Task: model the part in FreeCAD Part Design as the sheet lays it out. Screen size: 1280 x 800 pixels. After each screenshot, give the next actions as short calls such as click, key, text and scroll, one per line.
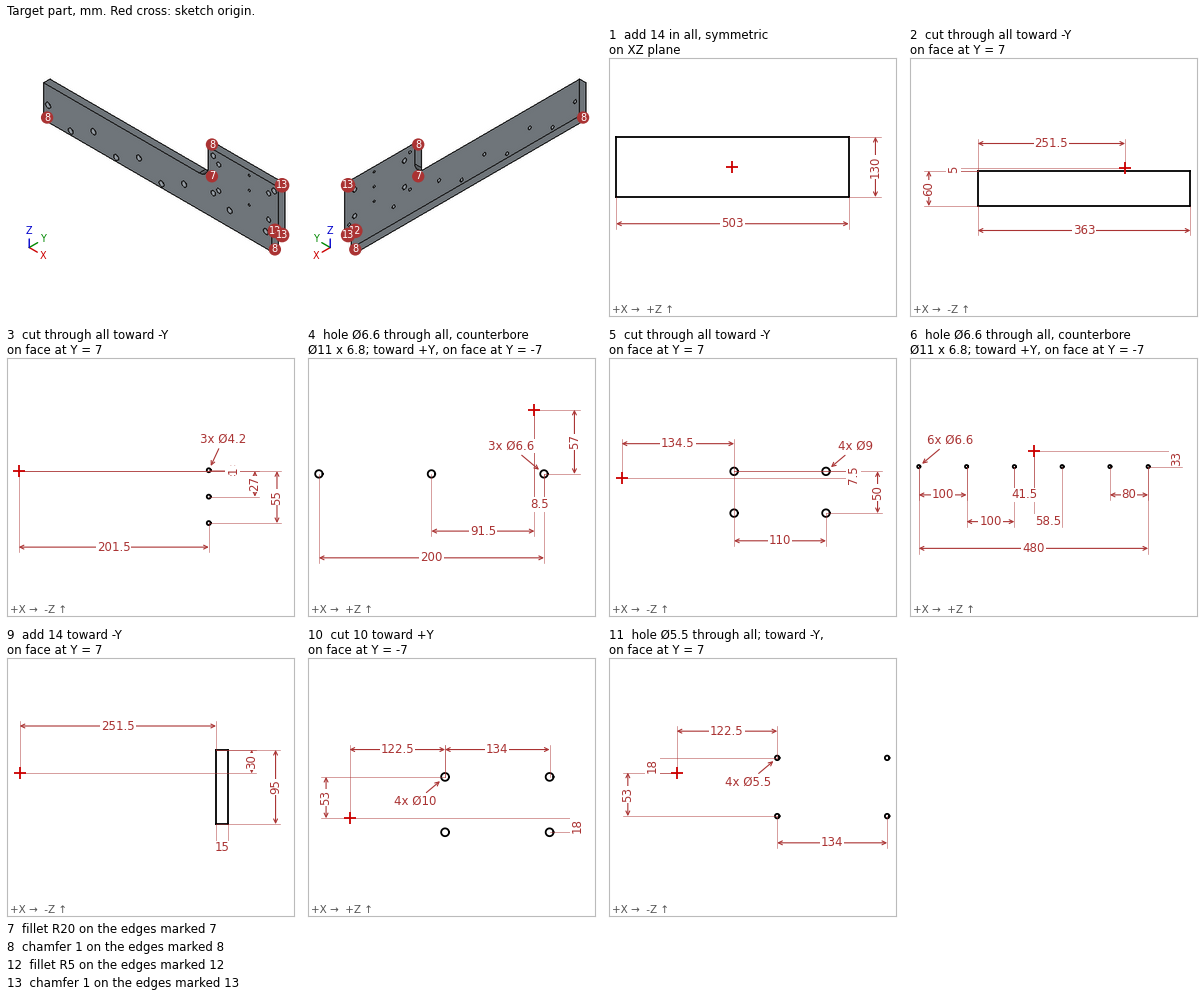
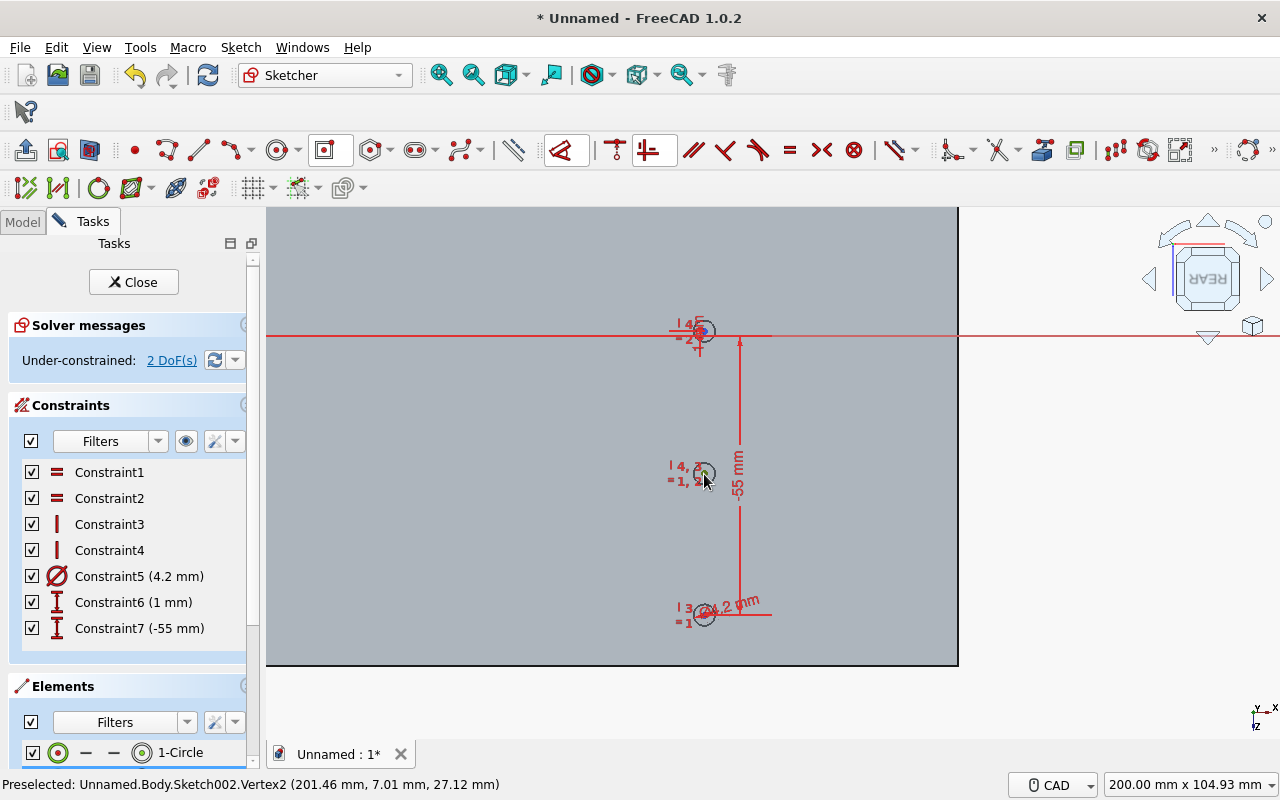
key(i)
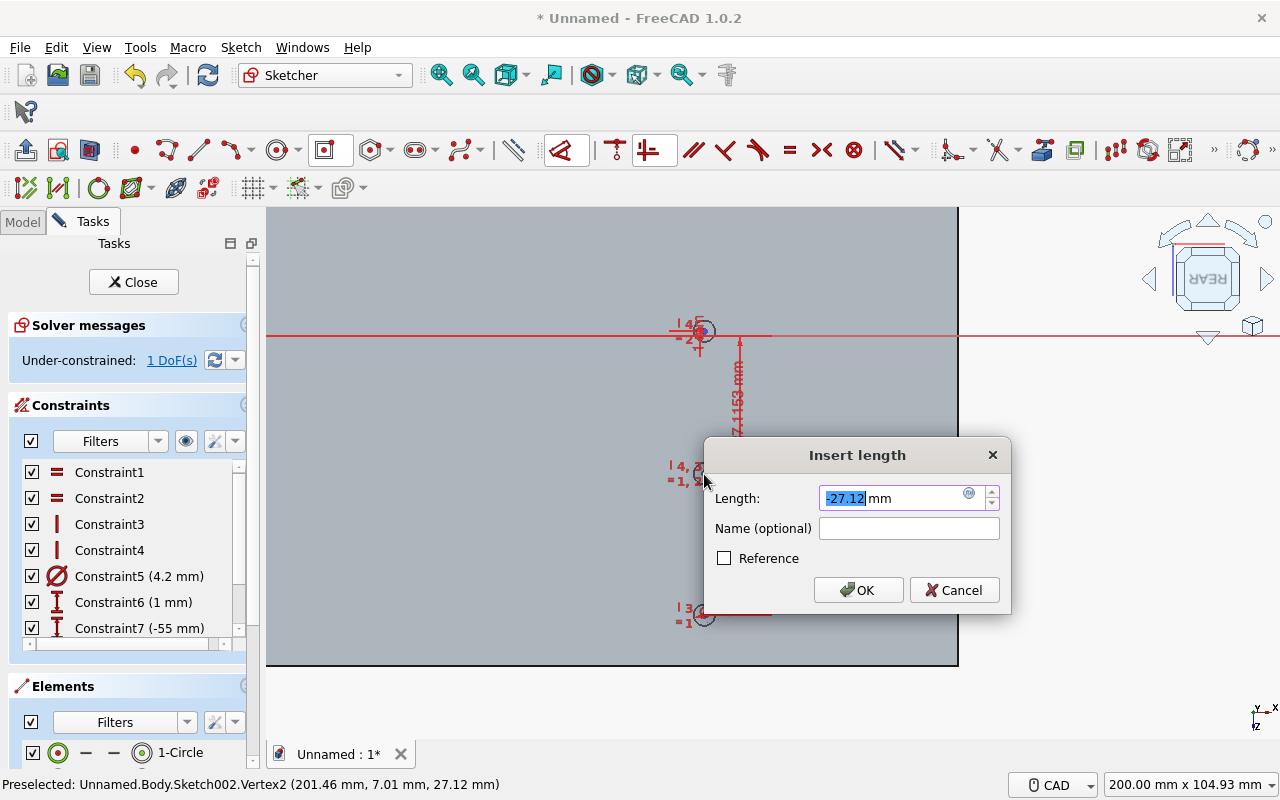
text(-27)
key(Return)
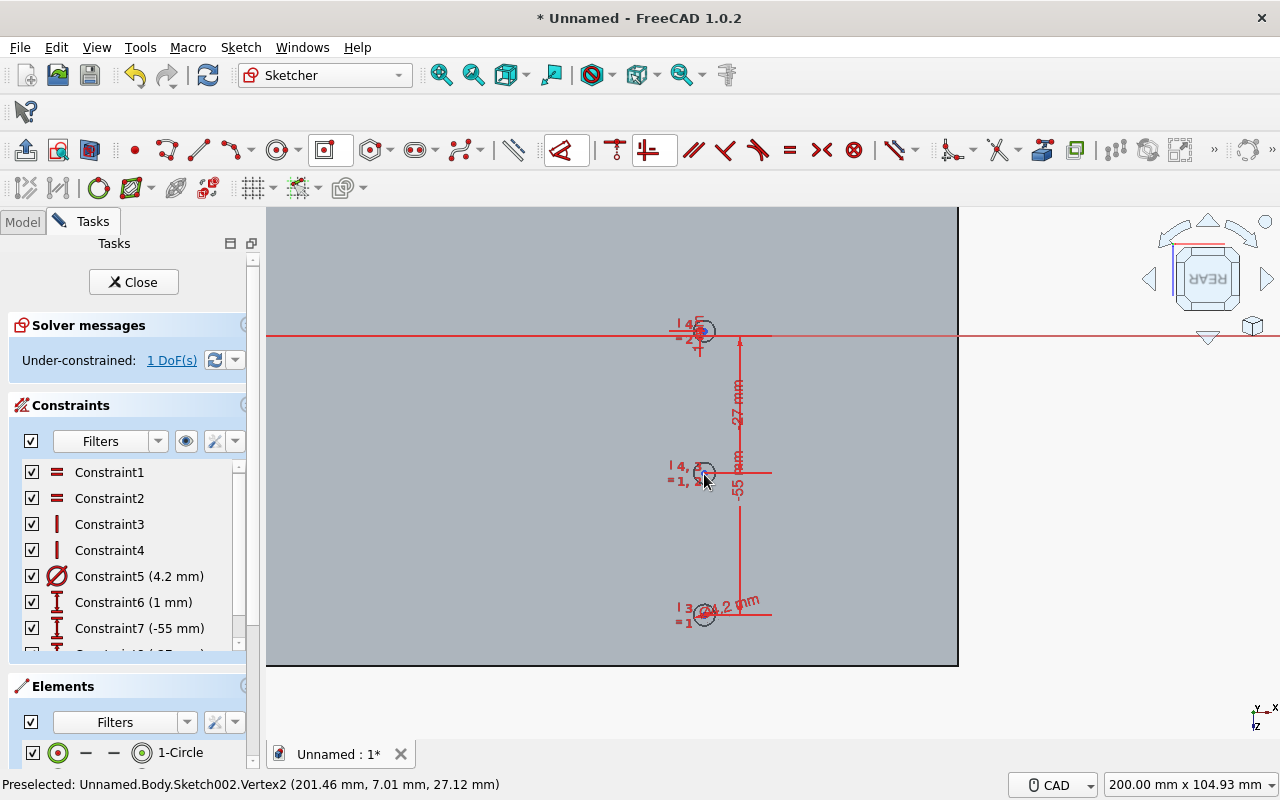
click(704, 615)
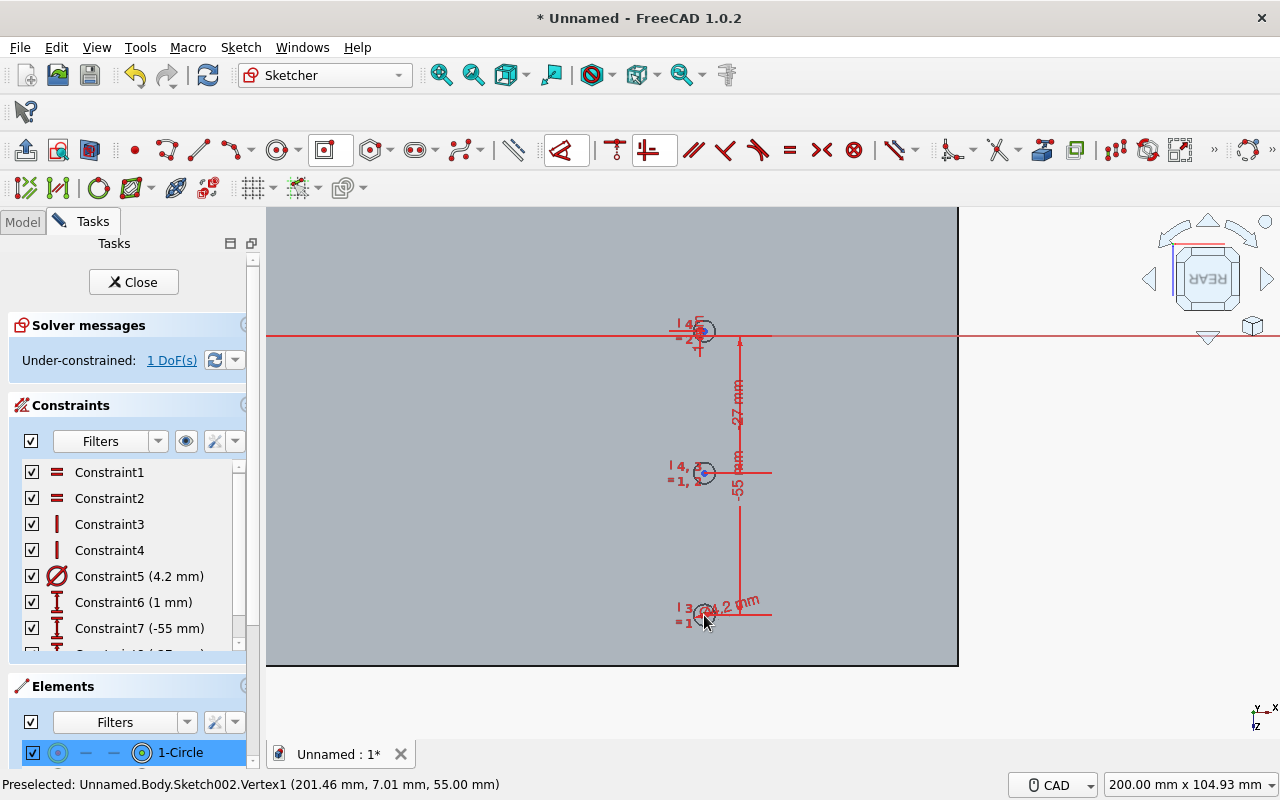
click(584, 150)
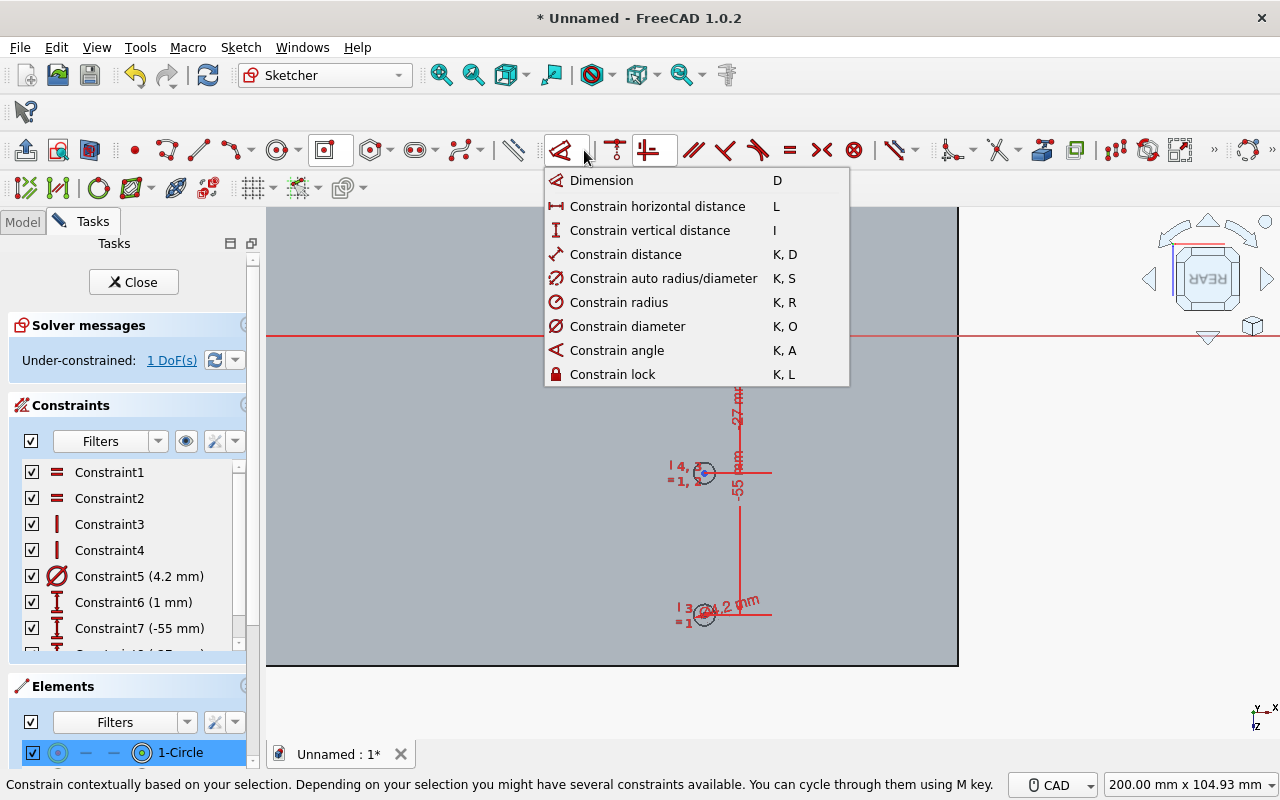
click(697, 206)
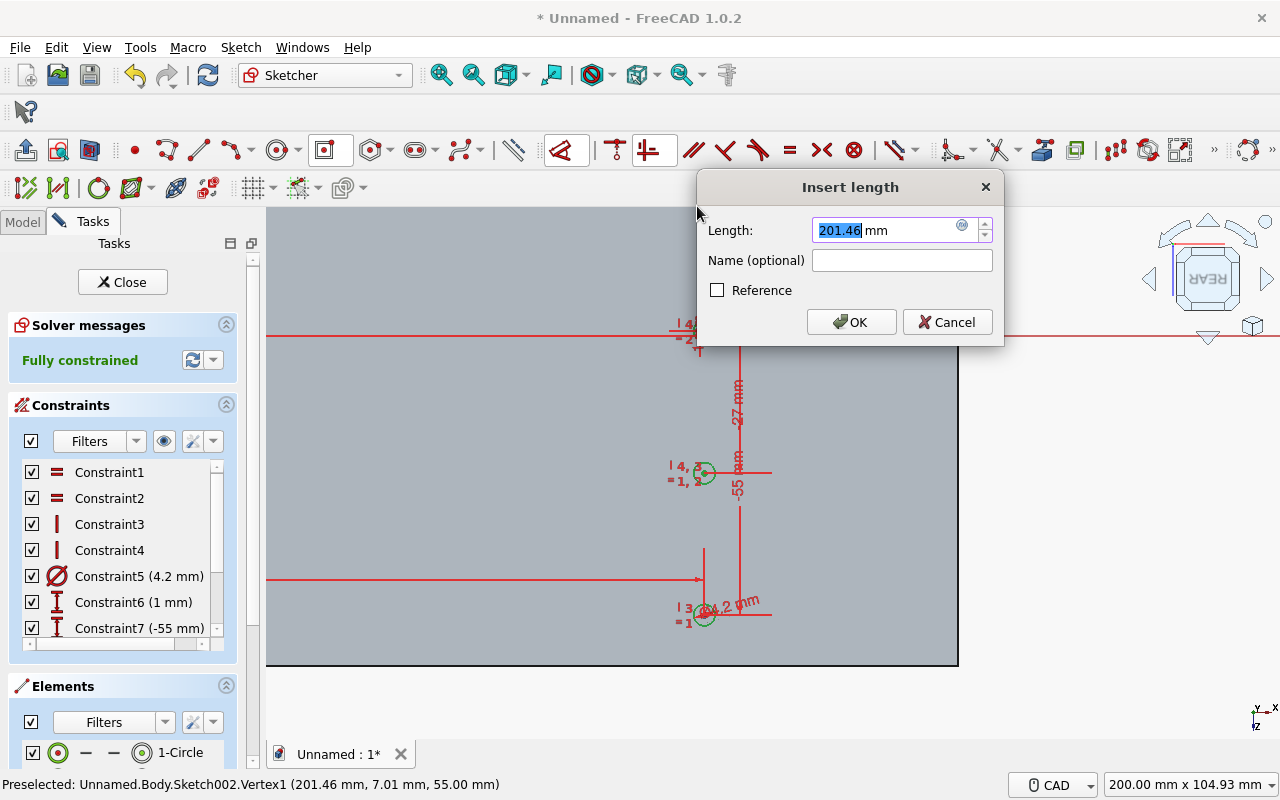
text(201.5)
key(Return)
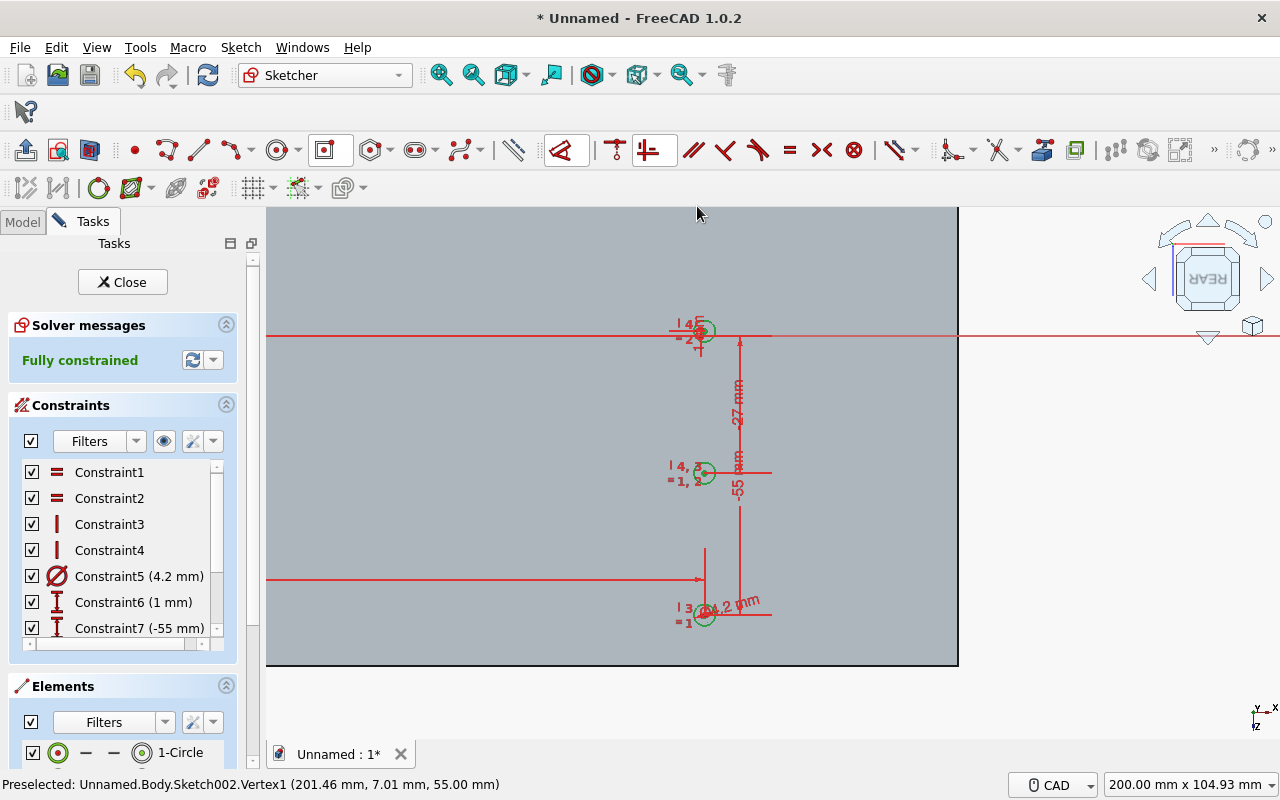
click(123, 282)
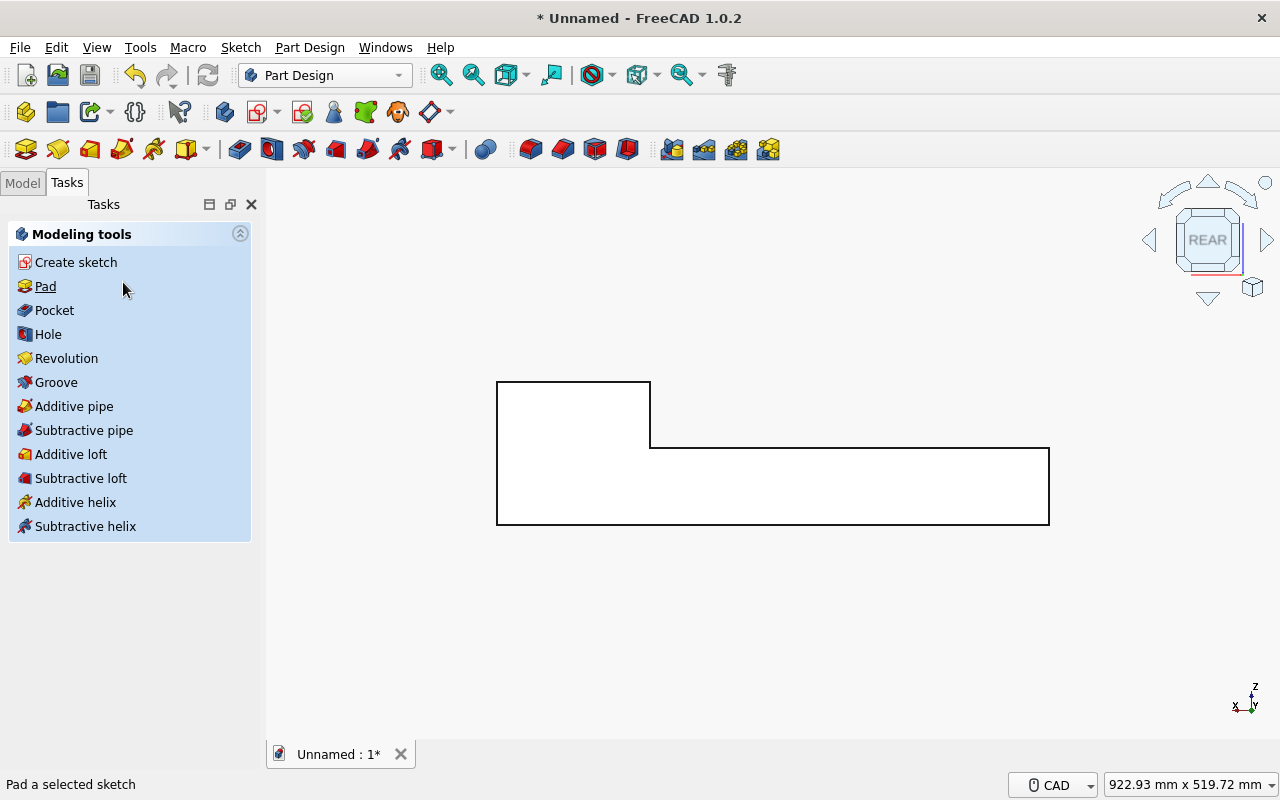
click(240, 150)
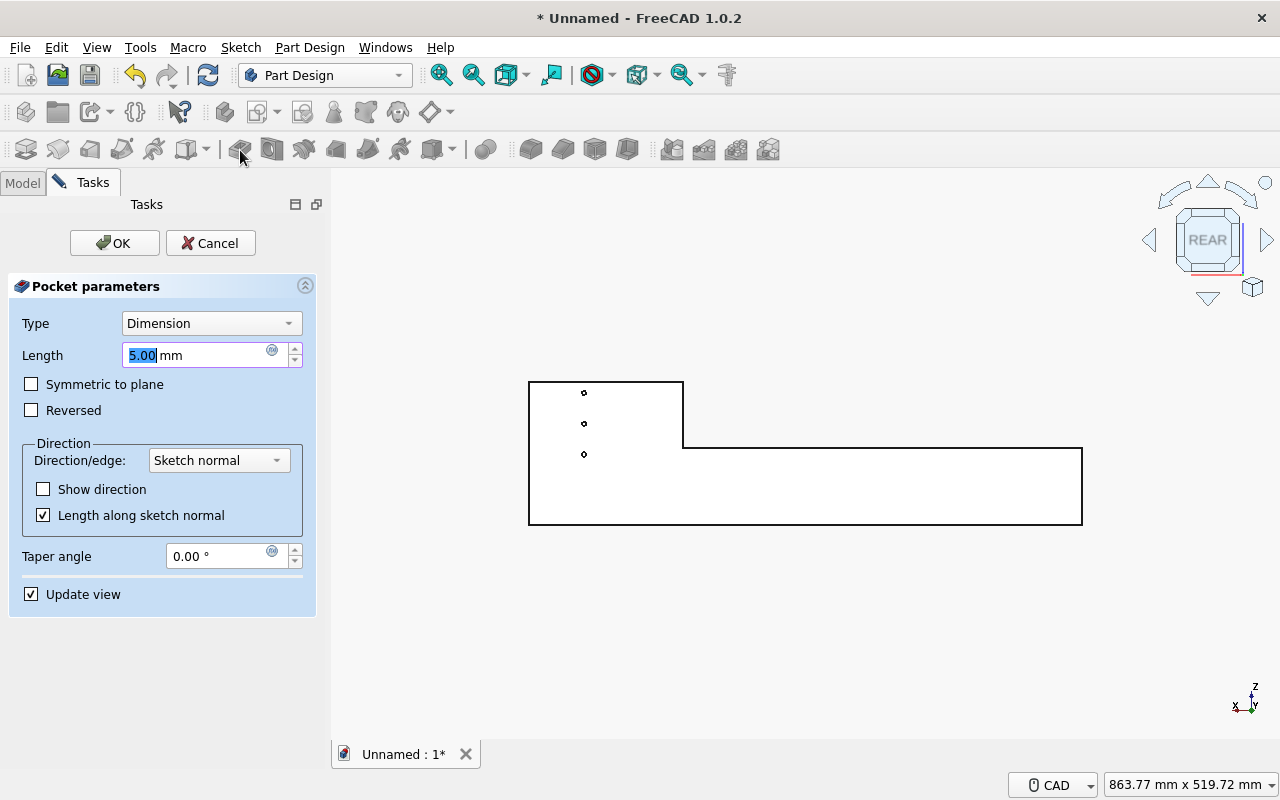
click(212, 324)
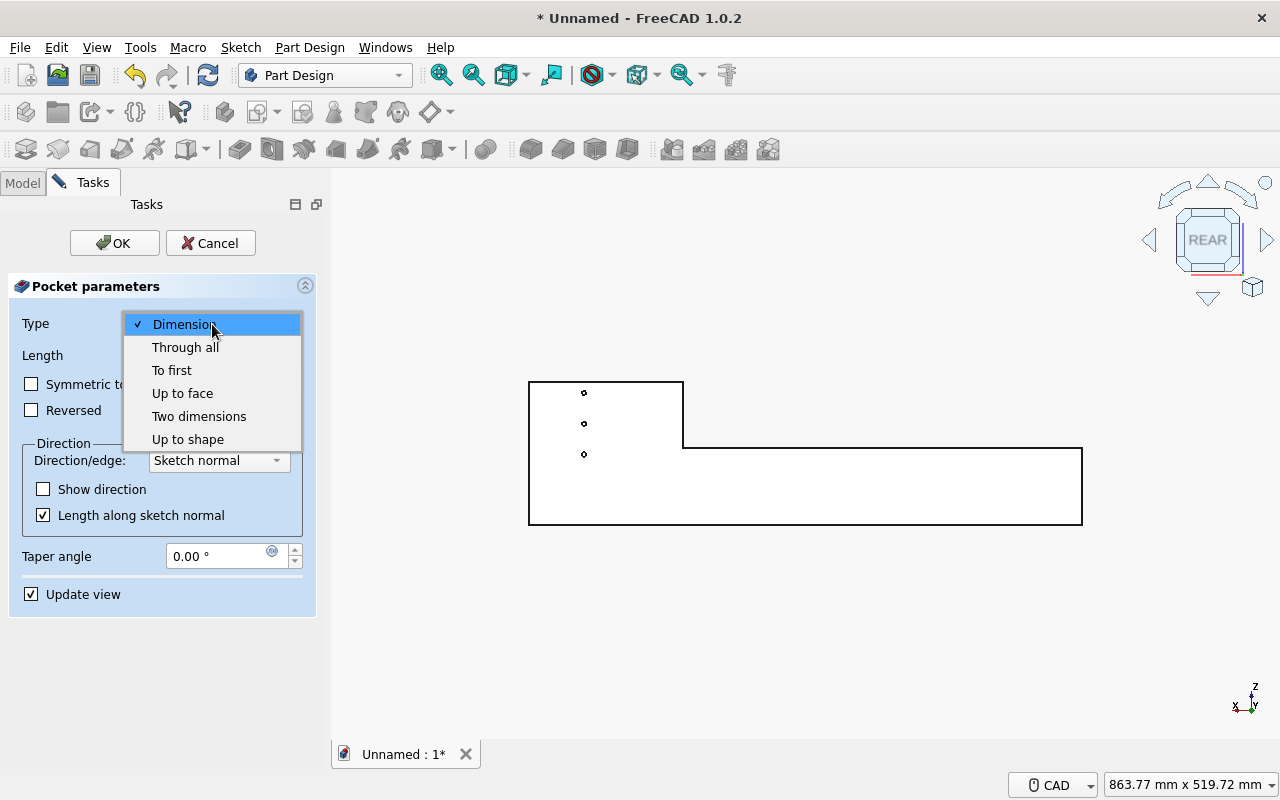
click(212, 348)